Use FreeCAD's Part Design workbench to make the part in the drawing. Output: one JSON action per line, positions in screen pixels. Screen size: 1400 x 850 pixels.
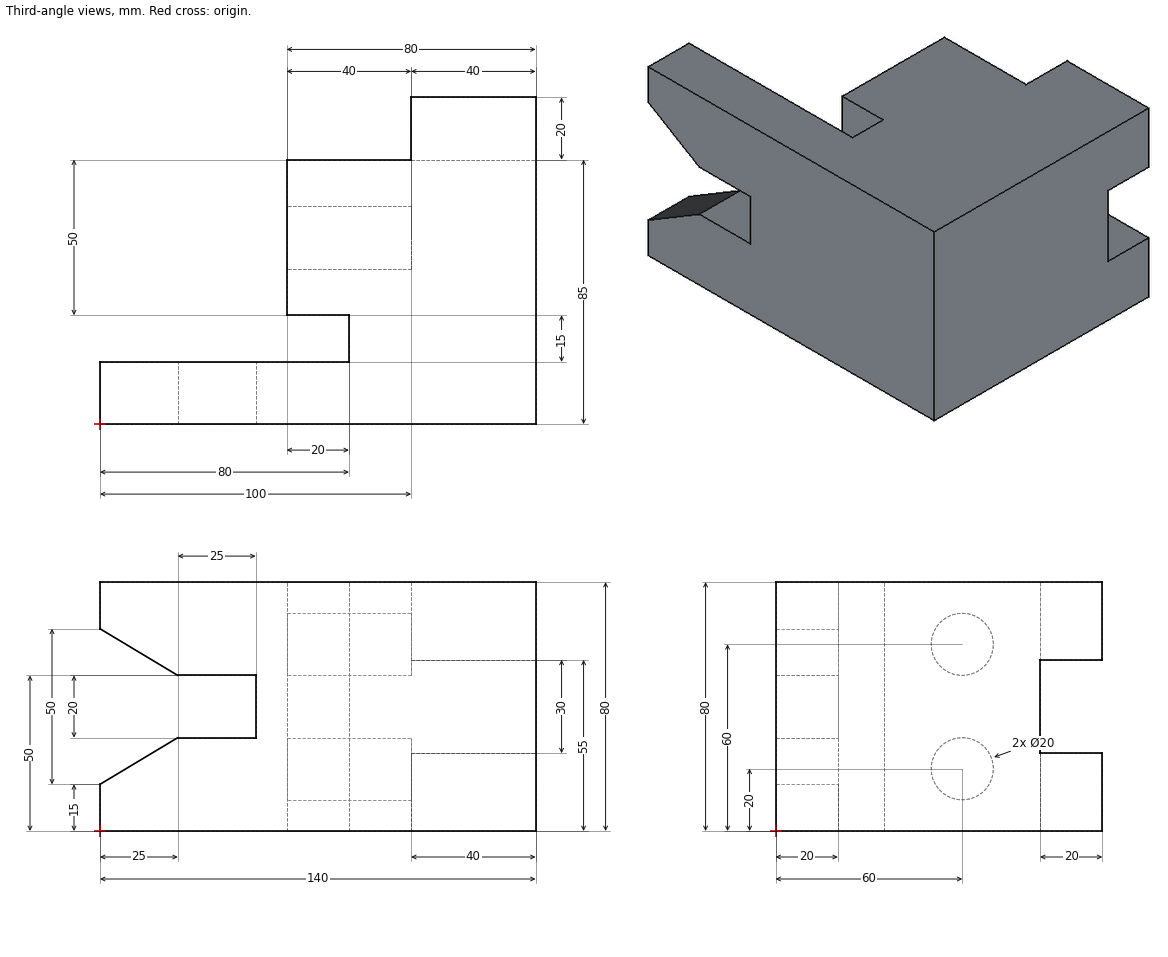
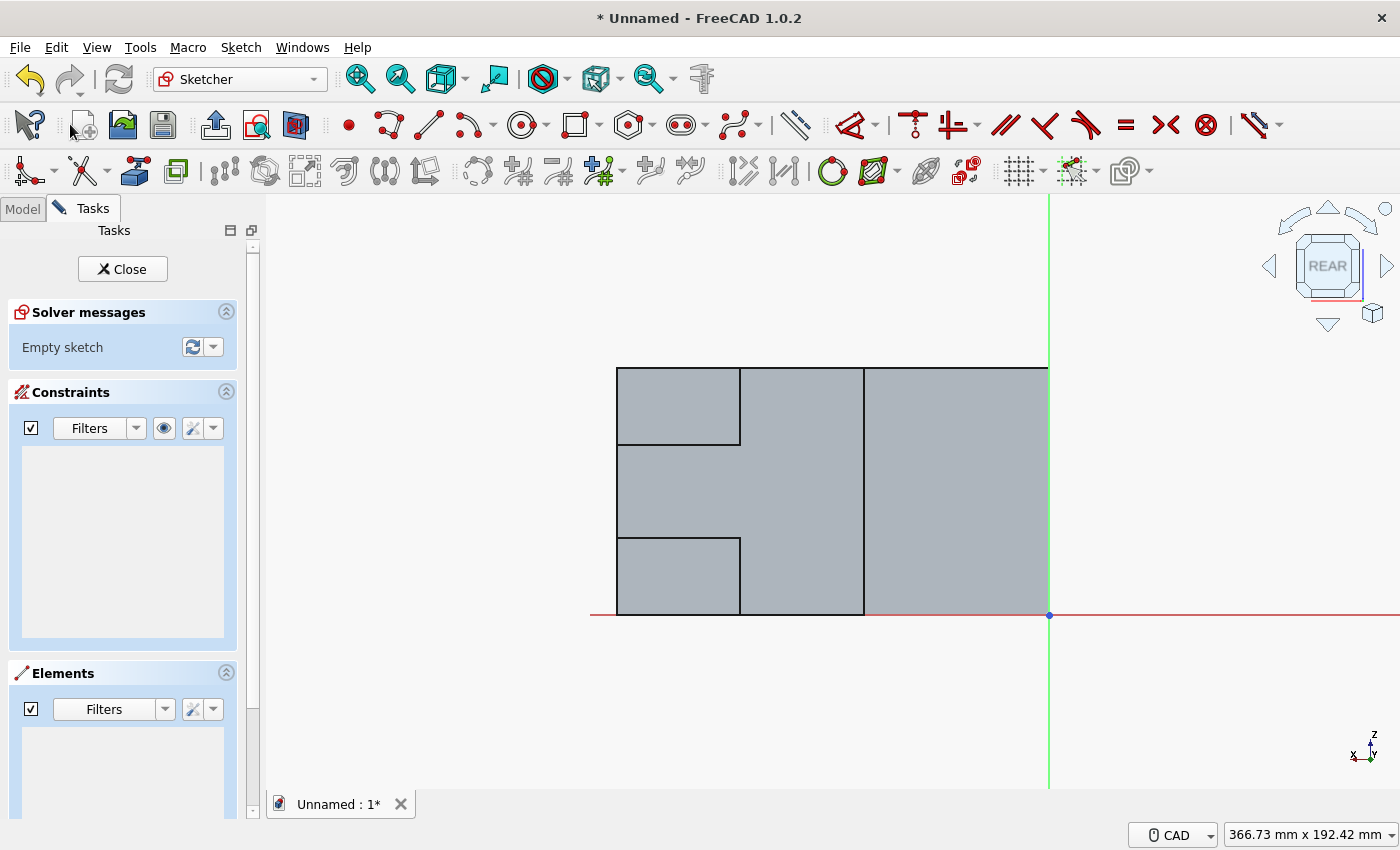
{"action": "left_click", "coordinate": [296, 126]}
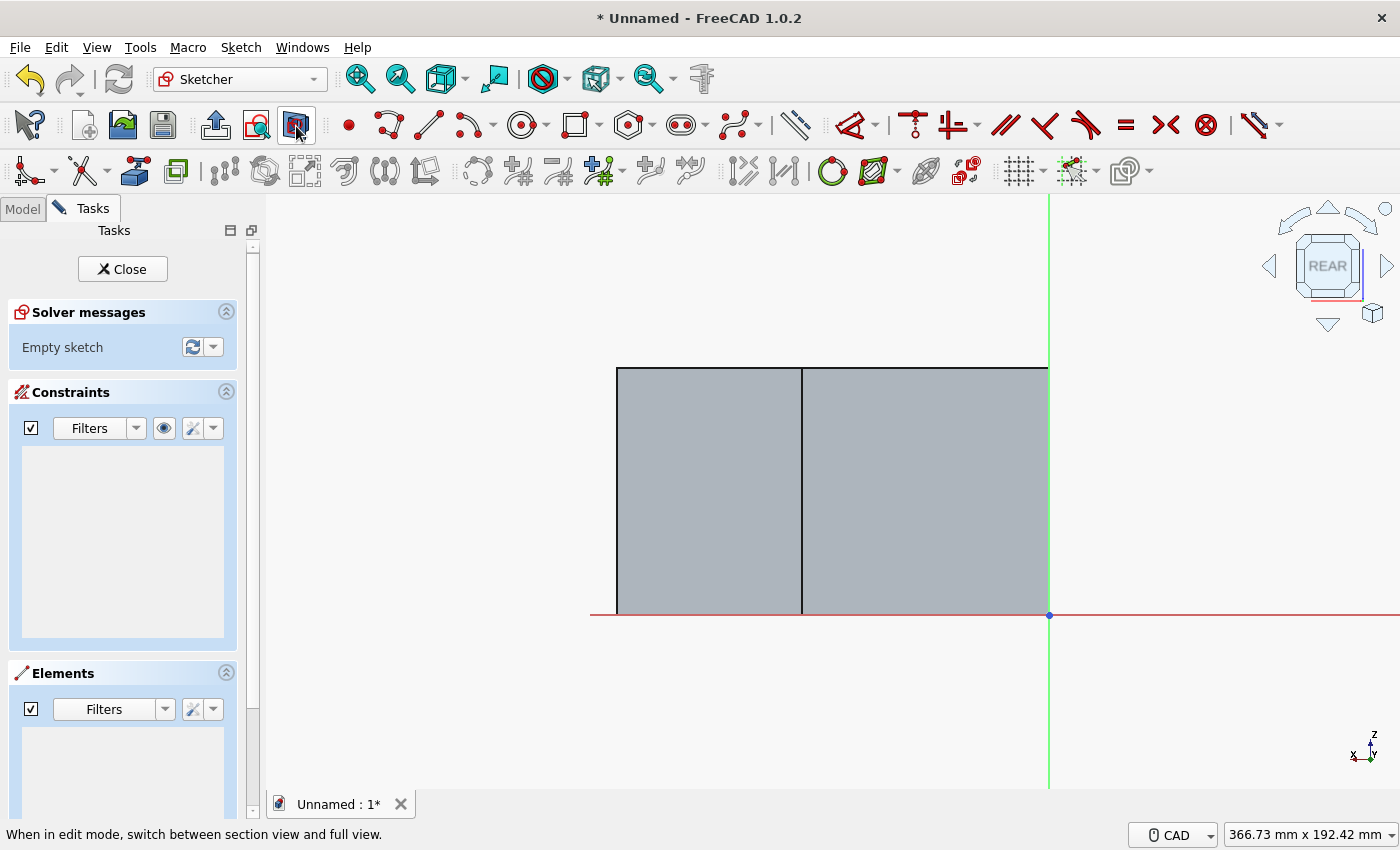
{"action": "scroll", "coordinate": [1225, 543], "scroll_direction": "up", "scroll_amount": 3}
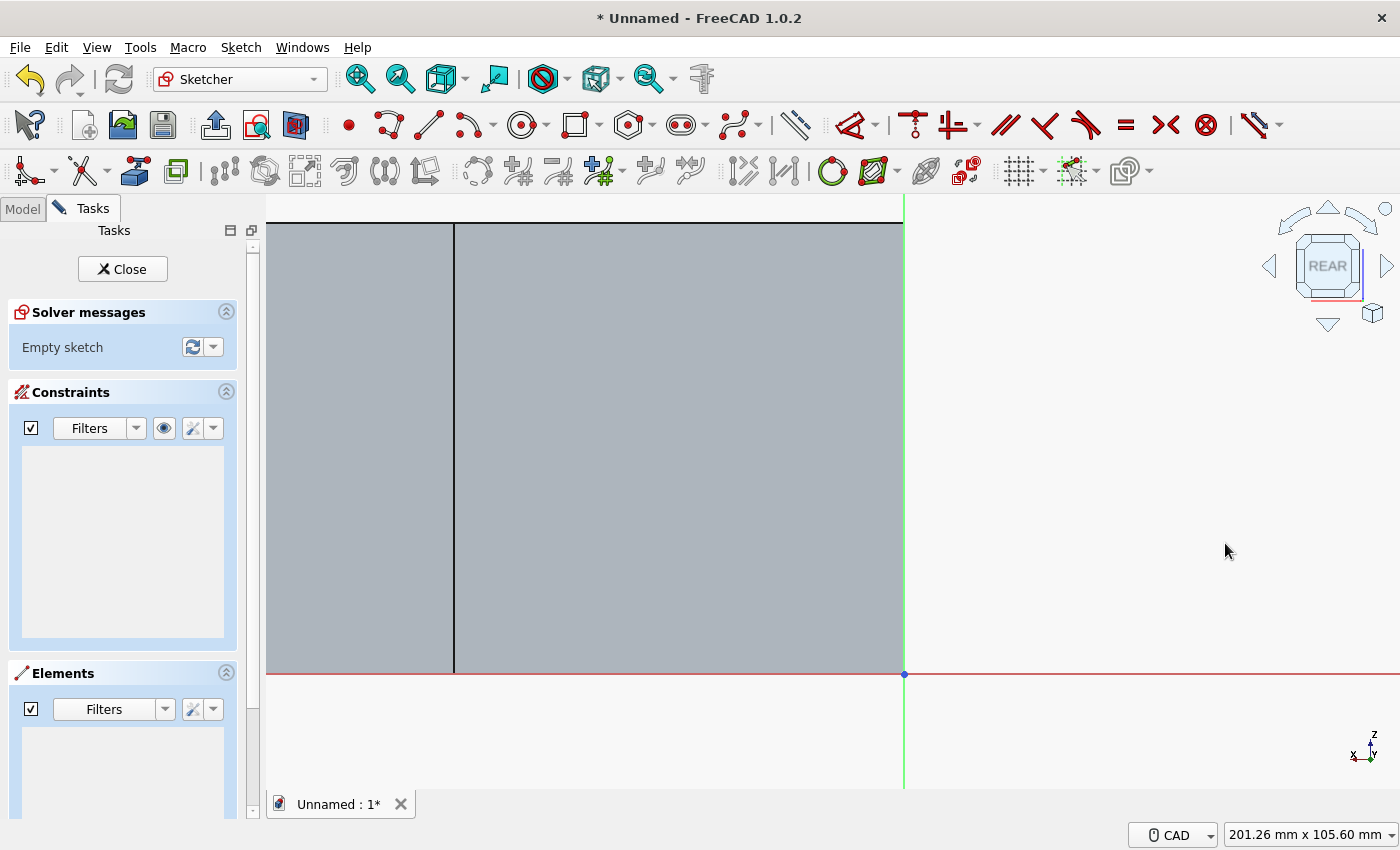
{"action": "key", "text": "g m"}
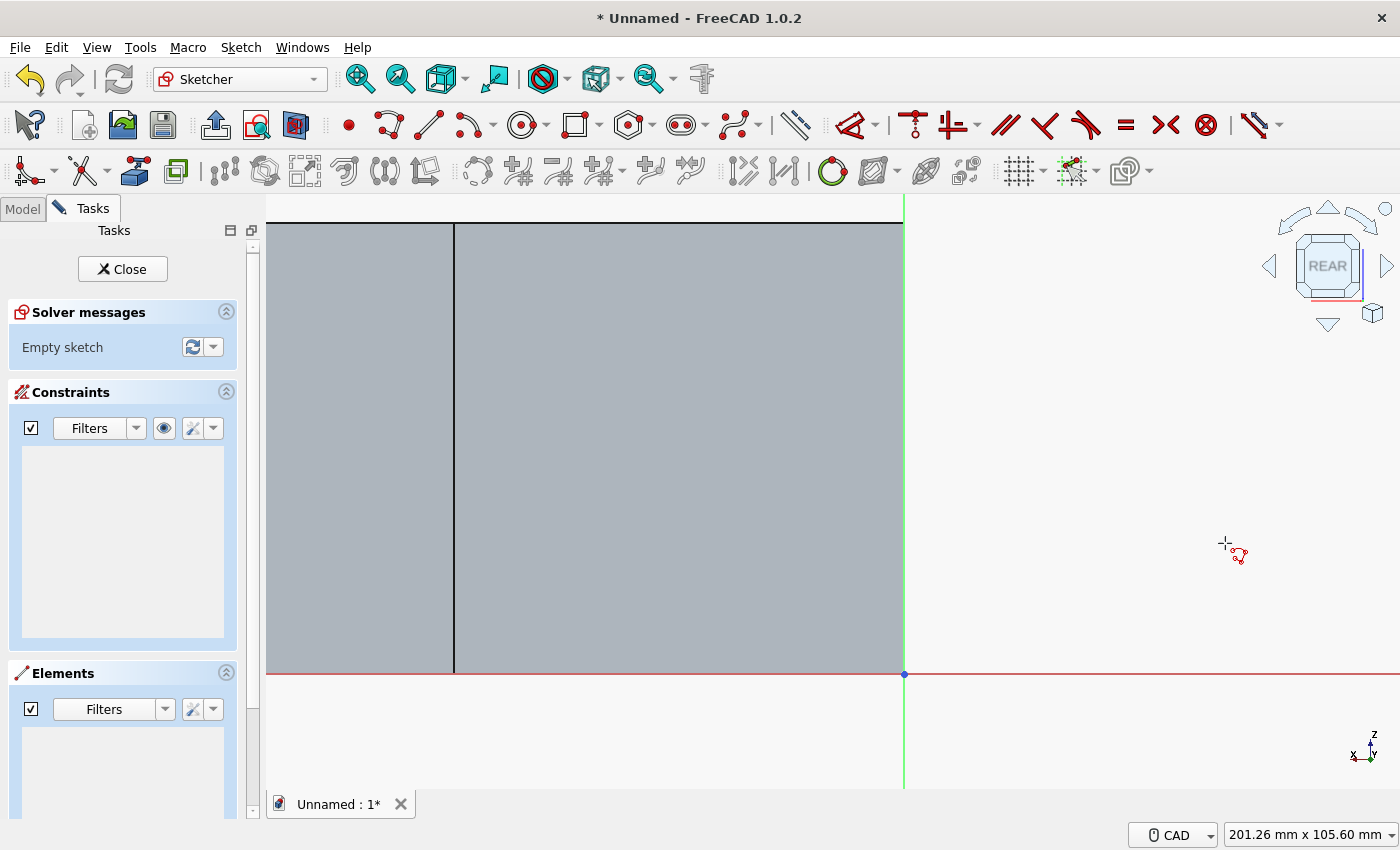
{"action": "left_click", "coordinate": [904, 590]}
{"action": "left_click", "coordinate": [895, 308]}
{"action": "left_click", "coordinate": [764, 392]}
{"action": "left_click", "coordinate": [623, 392]}
{"action": "left_click", "coordinate": [623, 505]}
{"action": "left_click", "coordinate": [764, 505]}
{"action": "left_click", "coordinate": [904, 591]}
{"action": "key", "text": "Escape"}
{"action": "key", "text": "Escape"}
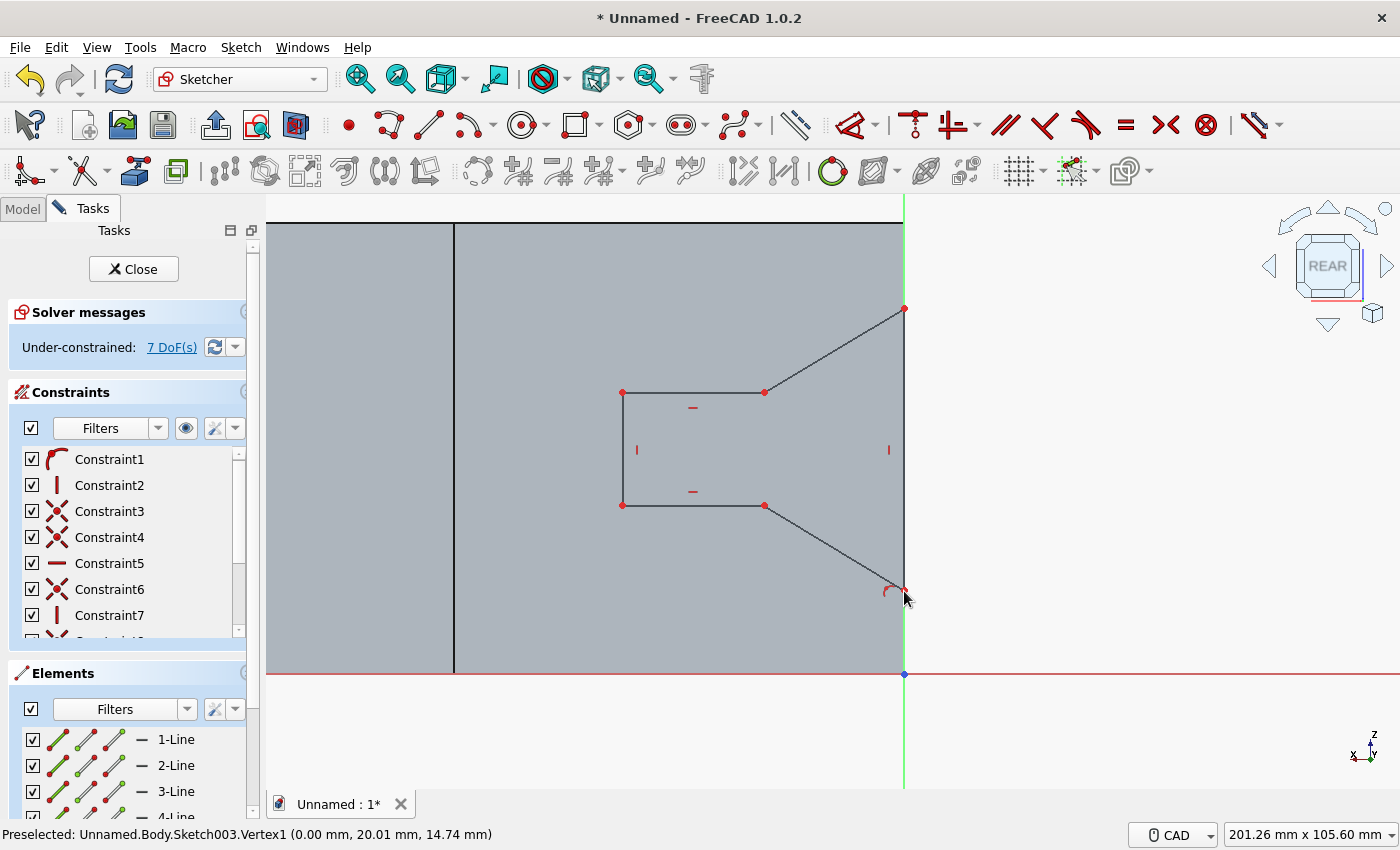
{"action": "left_click", "coordinate": [850, 126]}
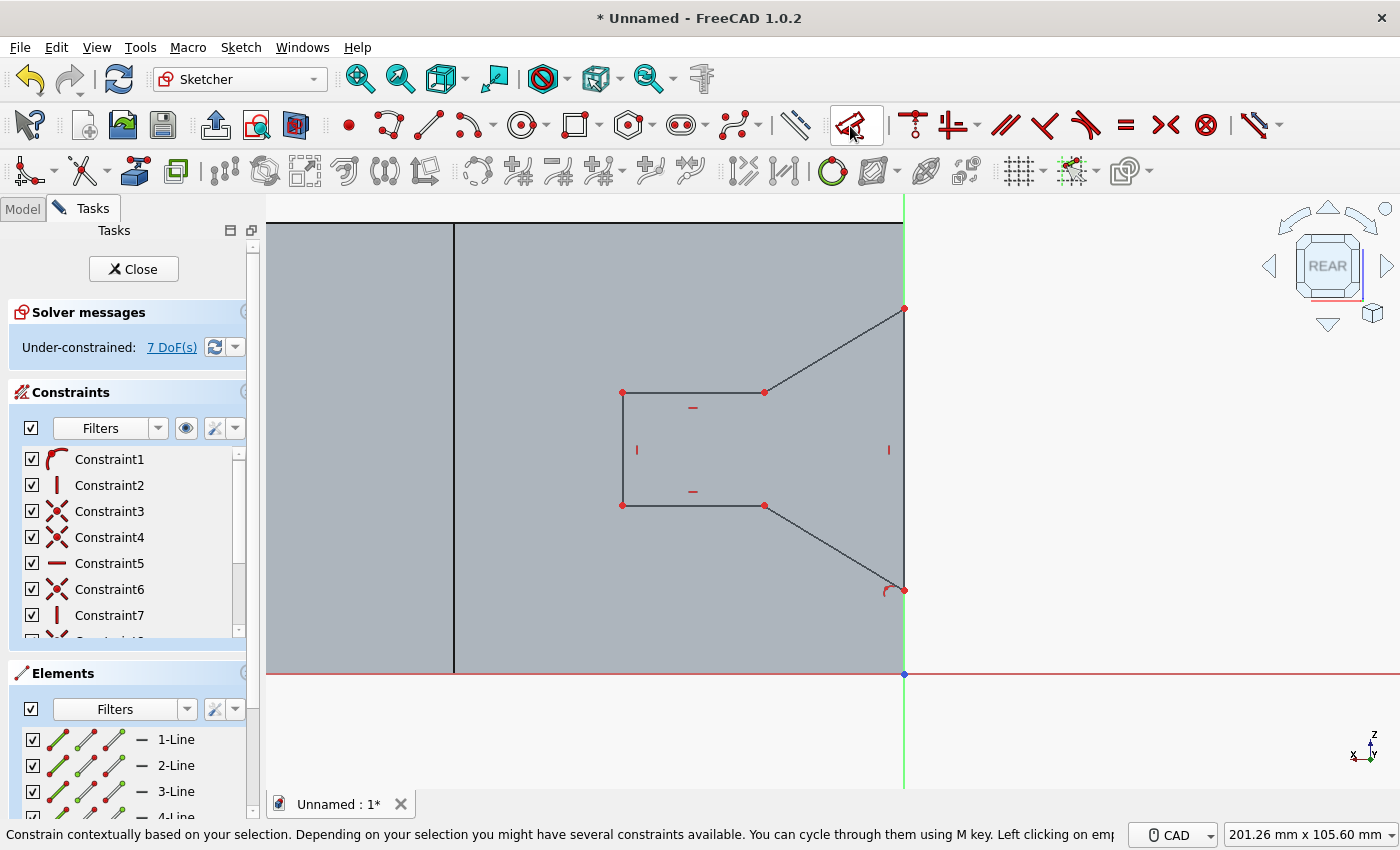
{"action": "left_click", "coordinate": [904, 506]}
{"action": "left_click", "coordinate": [938, 450]}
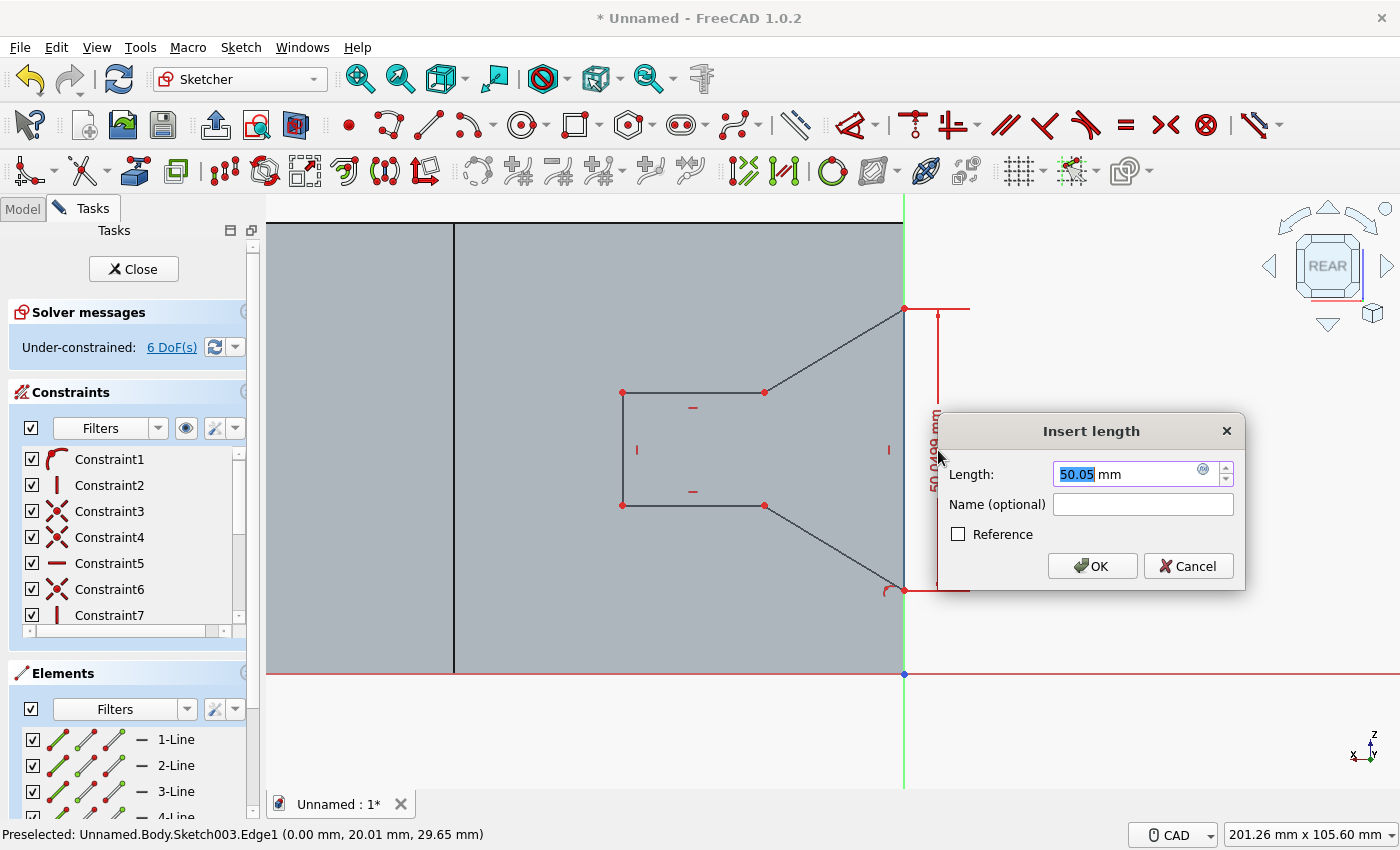
{"action": "type", "text": "50"}
{"action": "key", "text": "Return"}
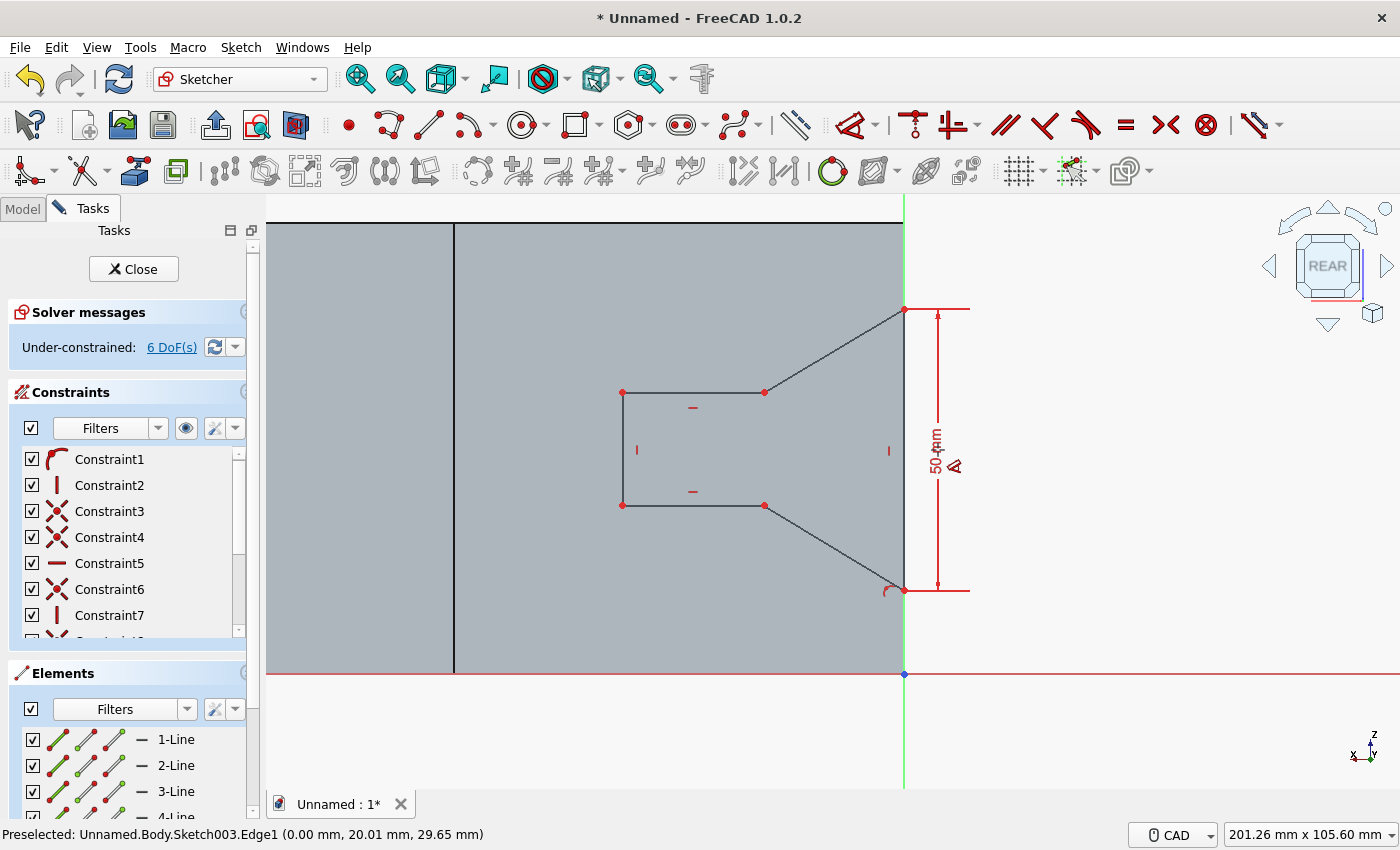
{"action": "left_click", "coordinate": [722, 393]}
{"action": "left_click", "coordinate": [693, 359]}